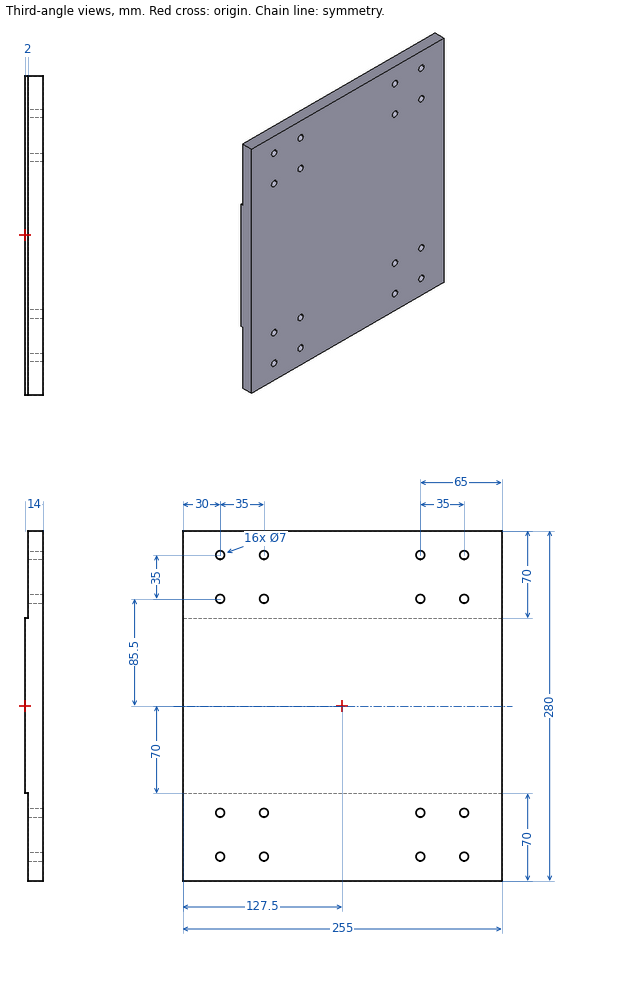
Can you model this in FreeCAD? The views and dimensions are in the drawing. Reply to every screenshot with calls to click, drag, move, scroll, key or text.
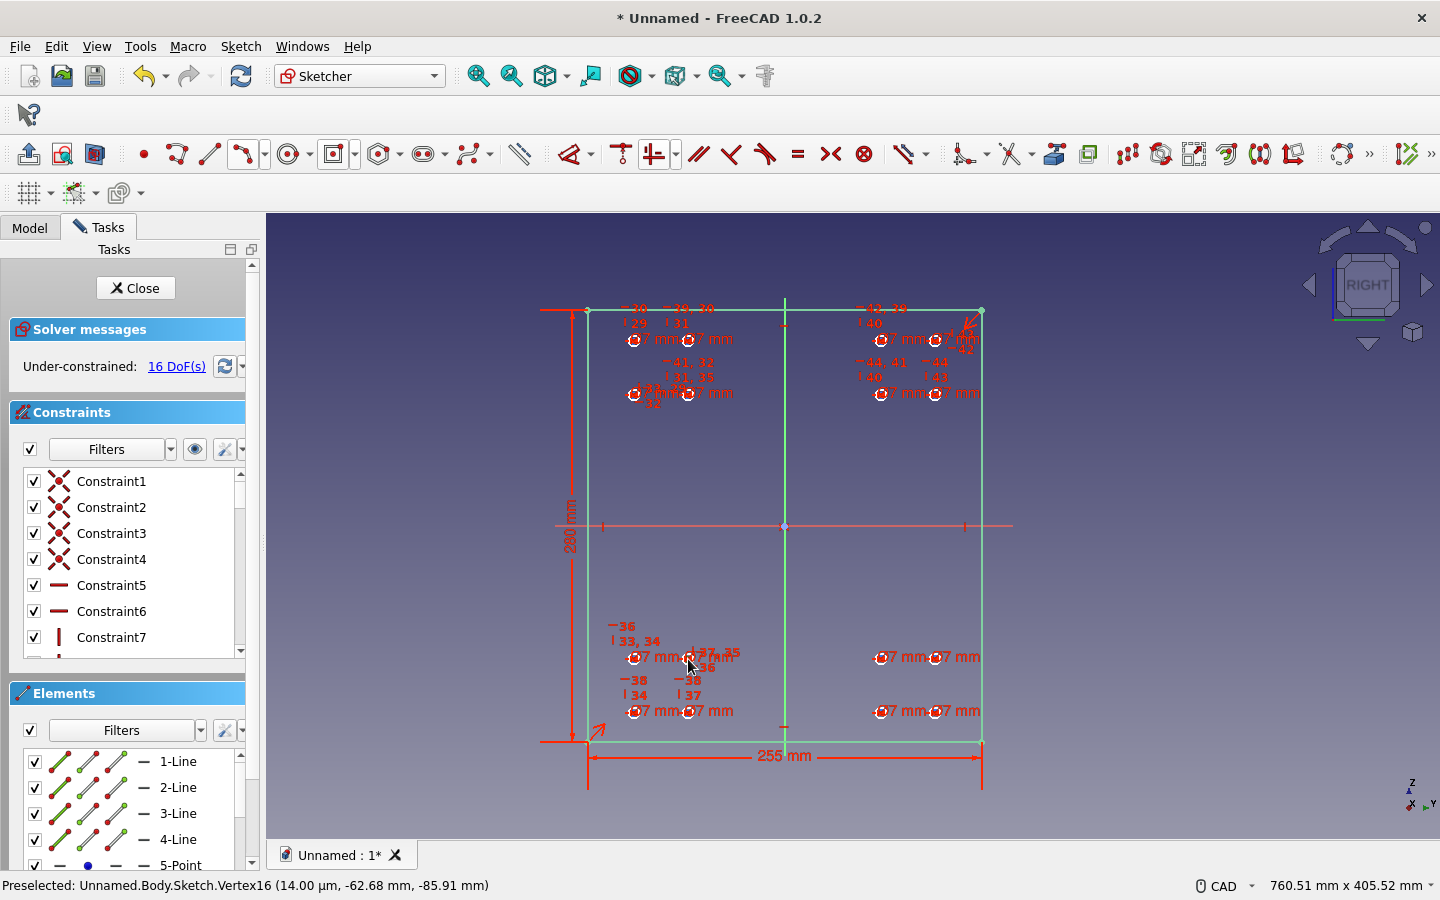
click(881, 659)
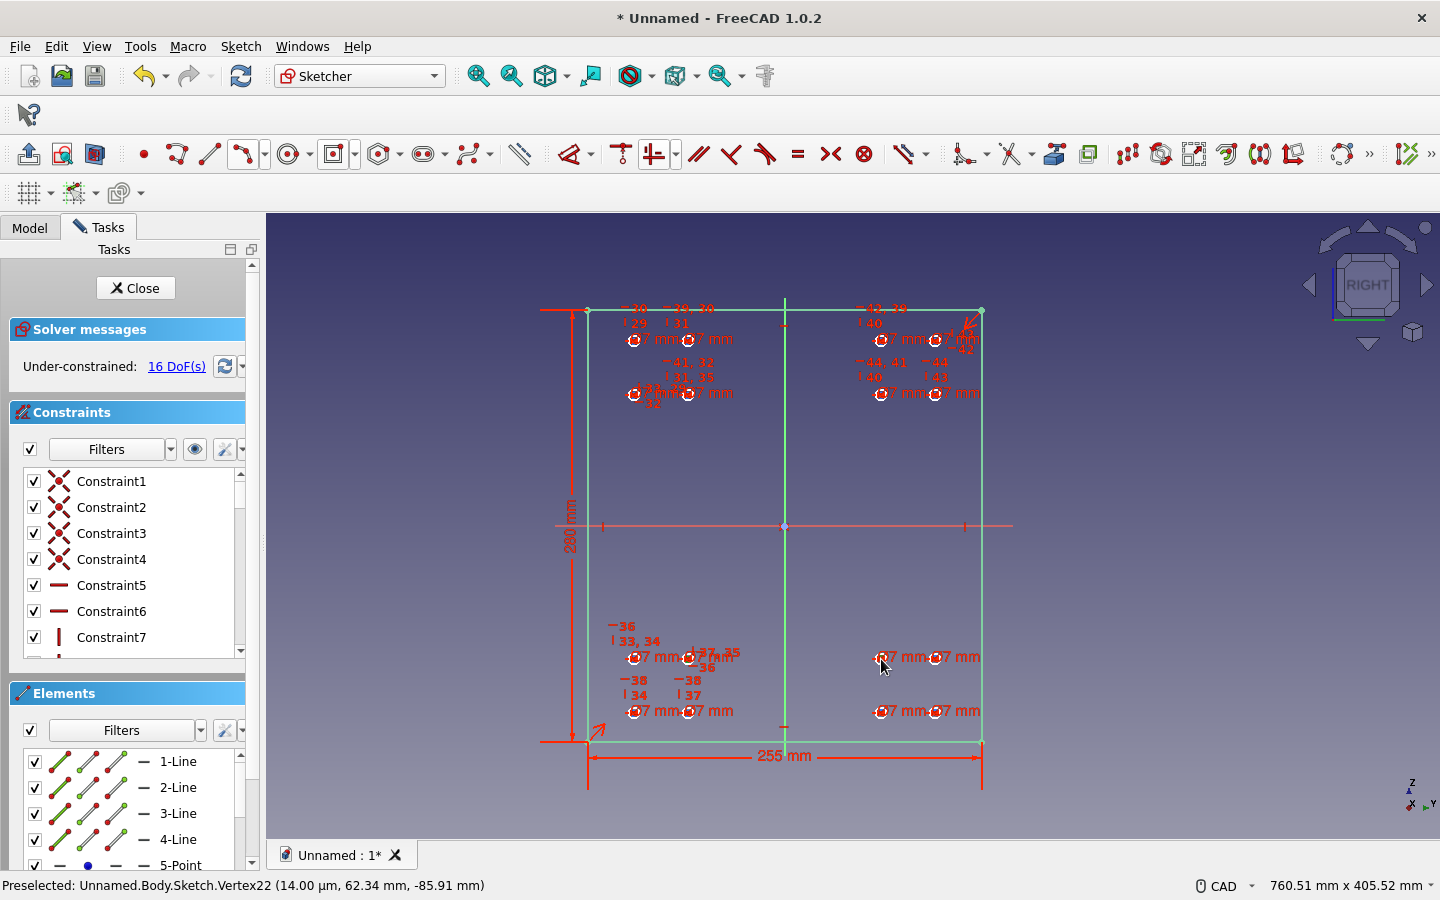
click(676, 154)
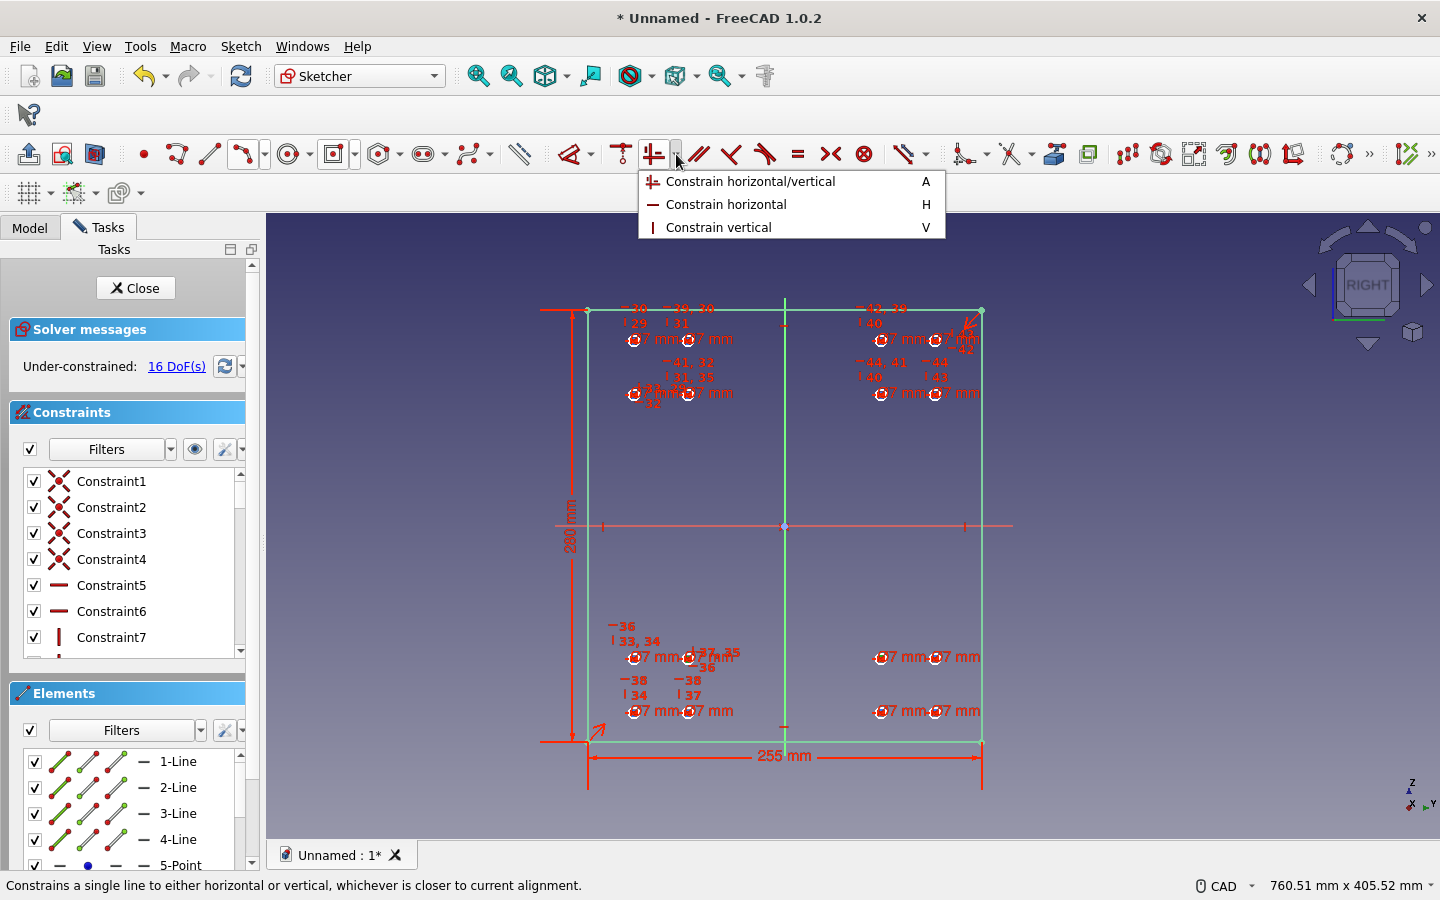
click(792, 204)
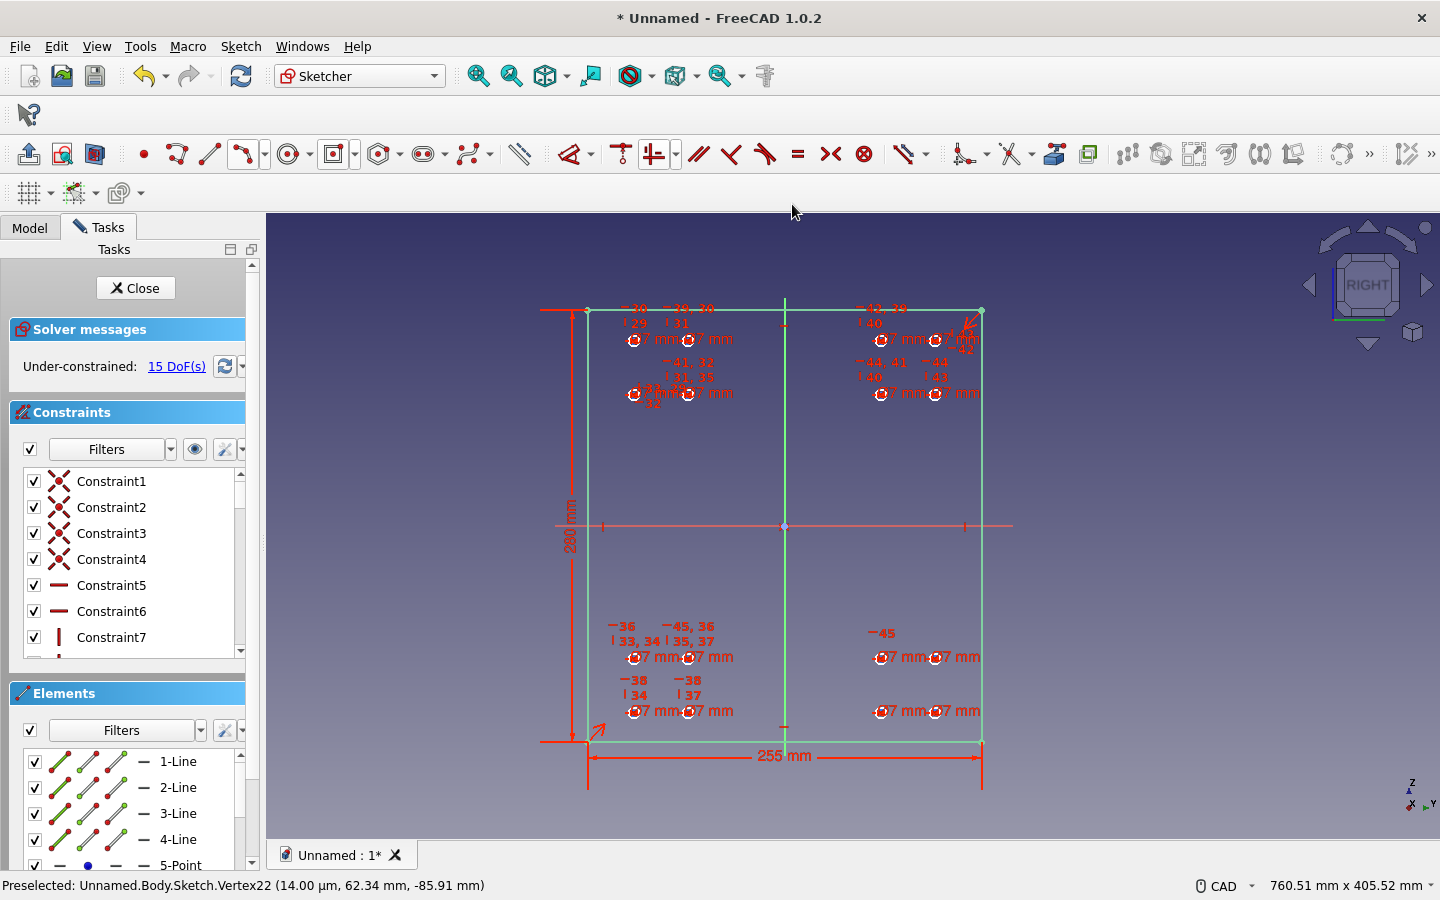
click(881, 659)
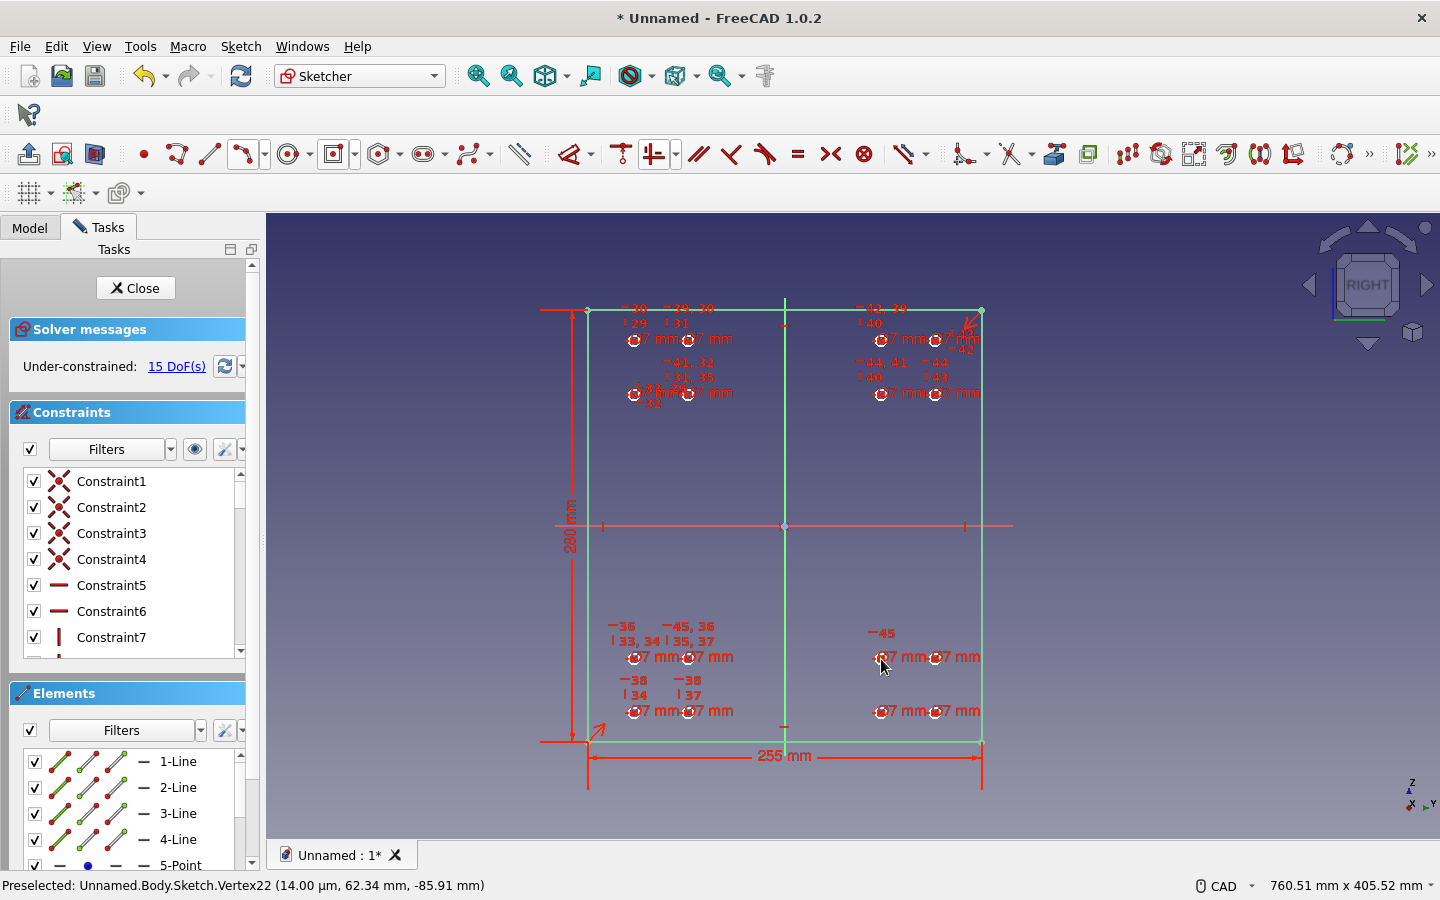
click(881, 713)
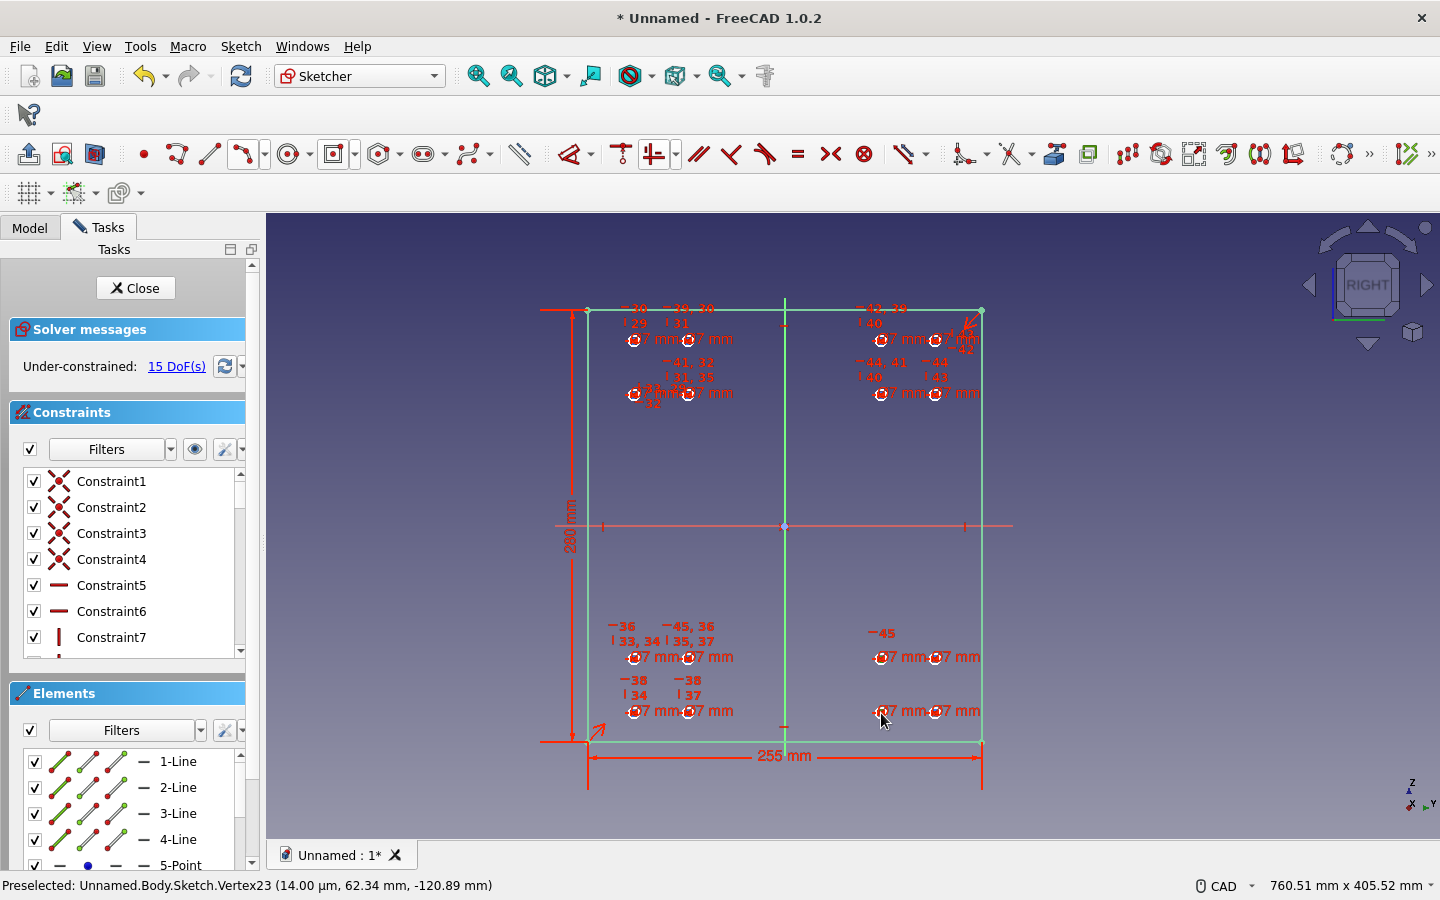
key(v)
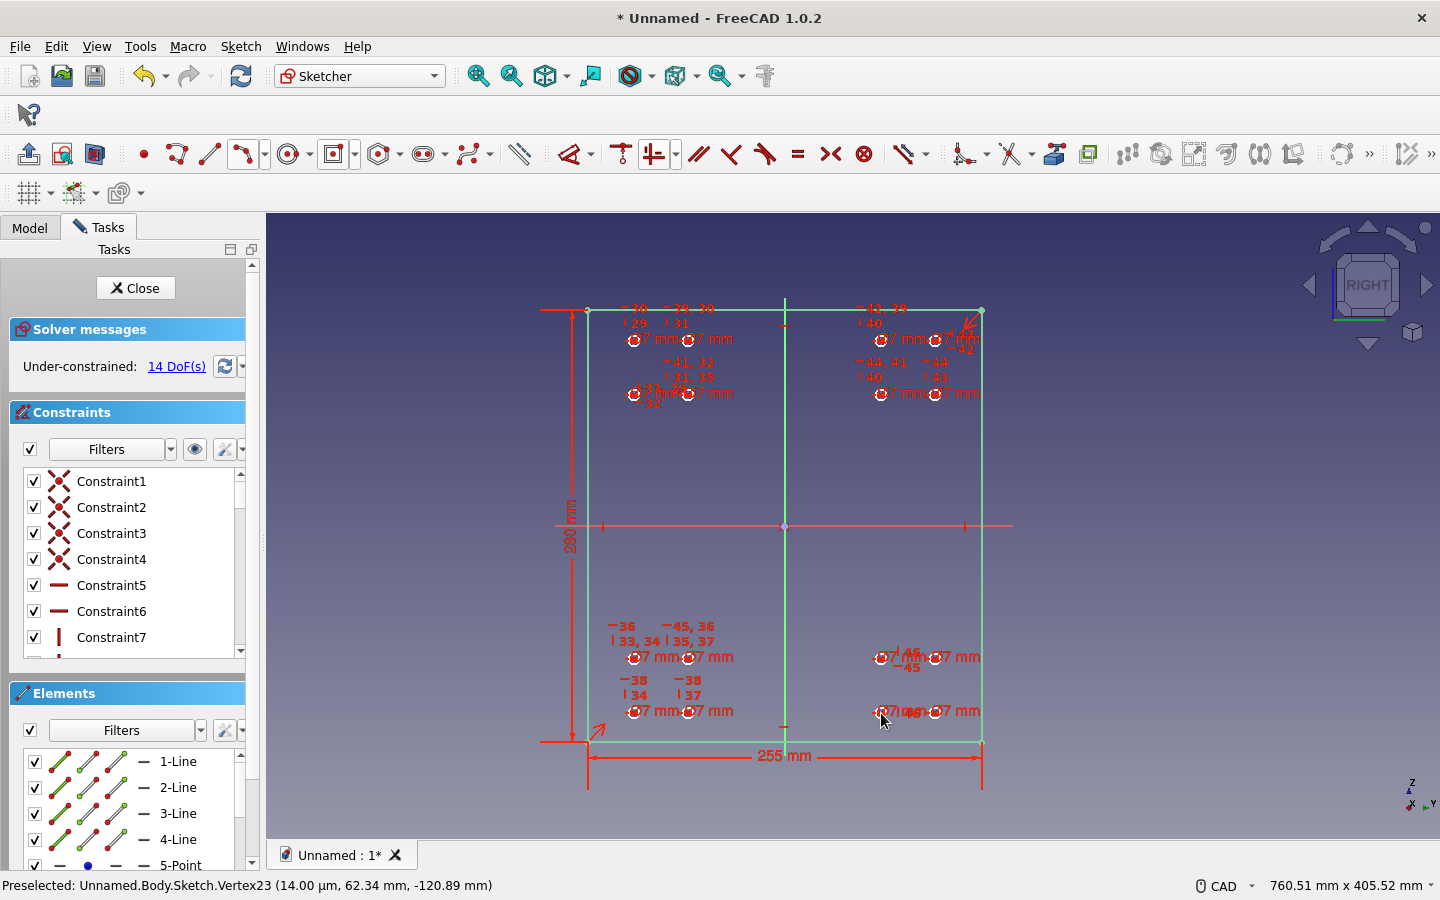
click(688, 713)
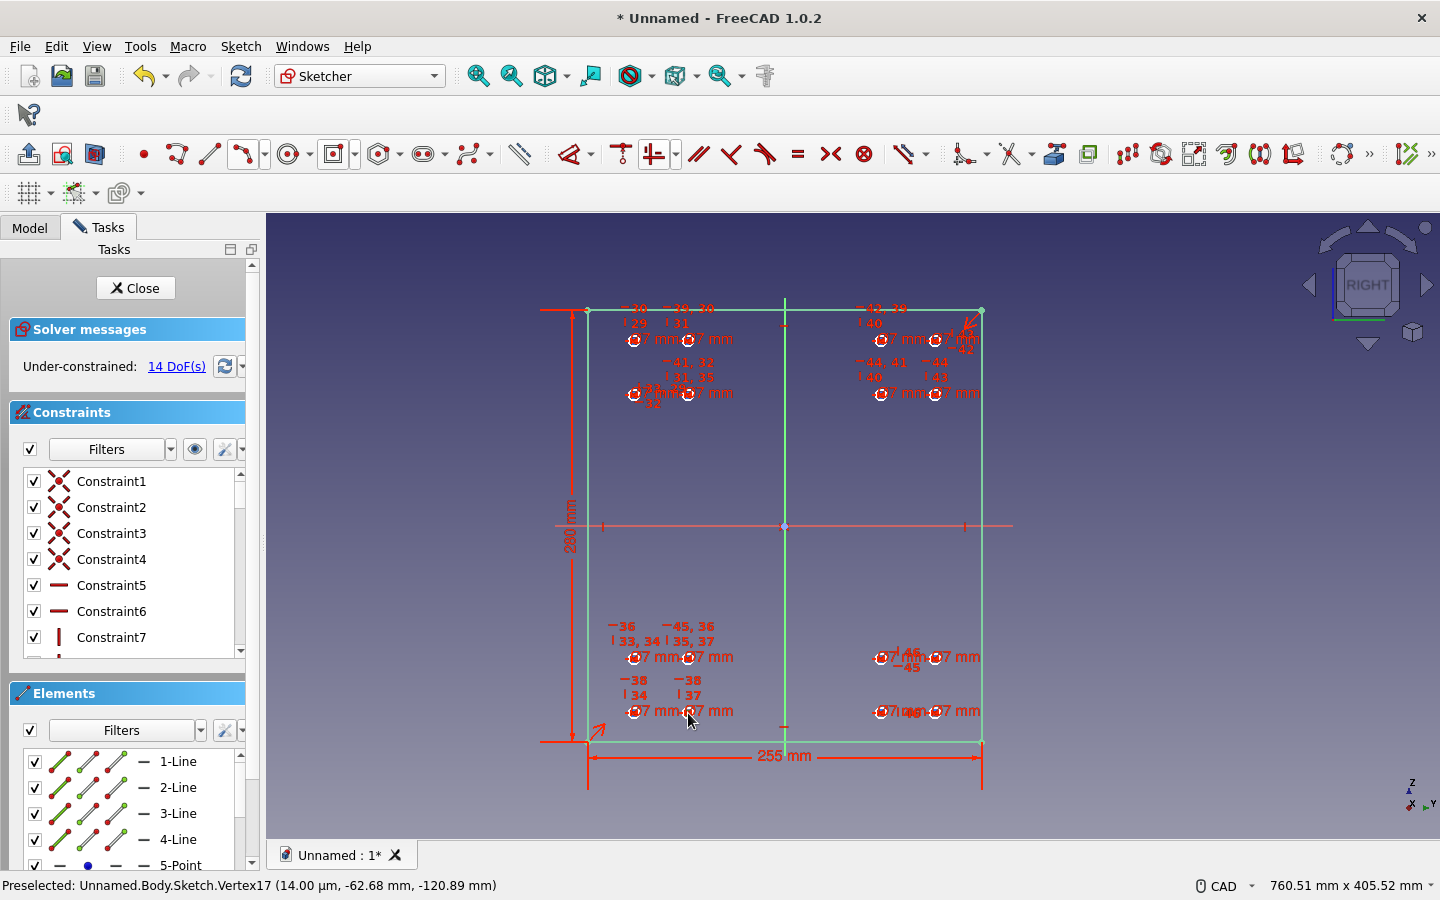
click(881, 713)